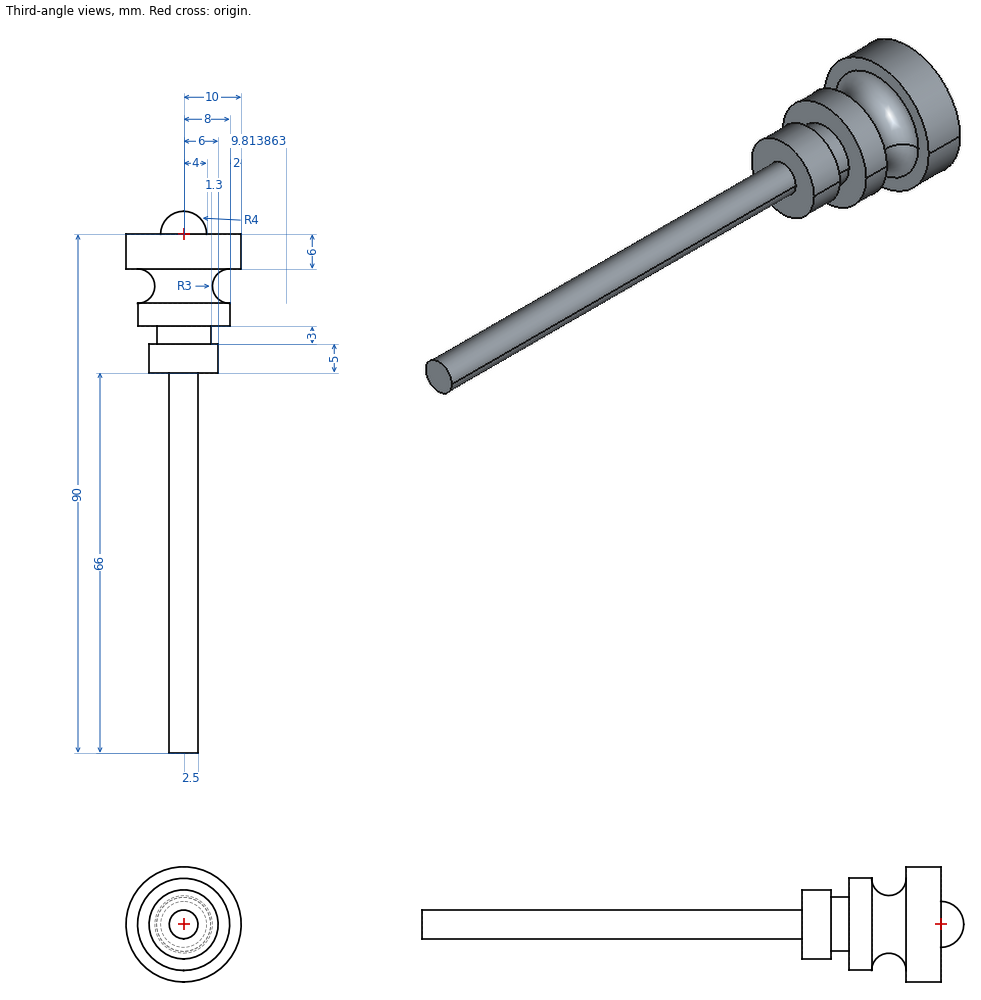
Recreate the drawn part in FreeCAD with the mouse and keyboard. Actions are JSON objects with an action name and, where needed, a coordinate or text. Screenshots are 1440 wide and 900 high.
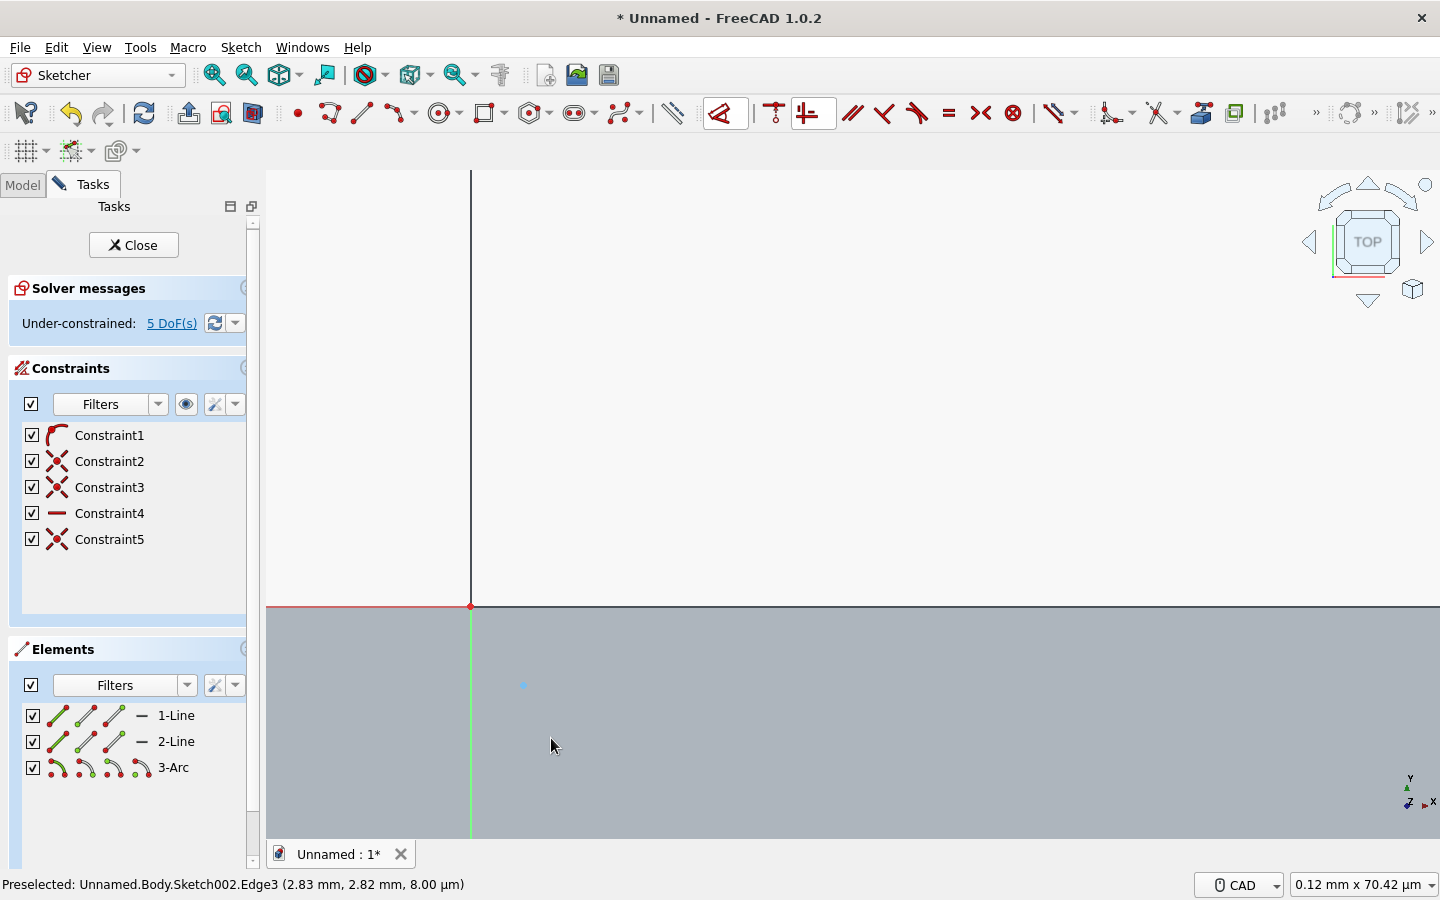
{"action": "left_click_drag", "start_coordinate": [461, 597], "coordinate": [533, 695]}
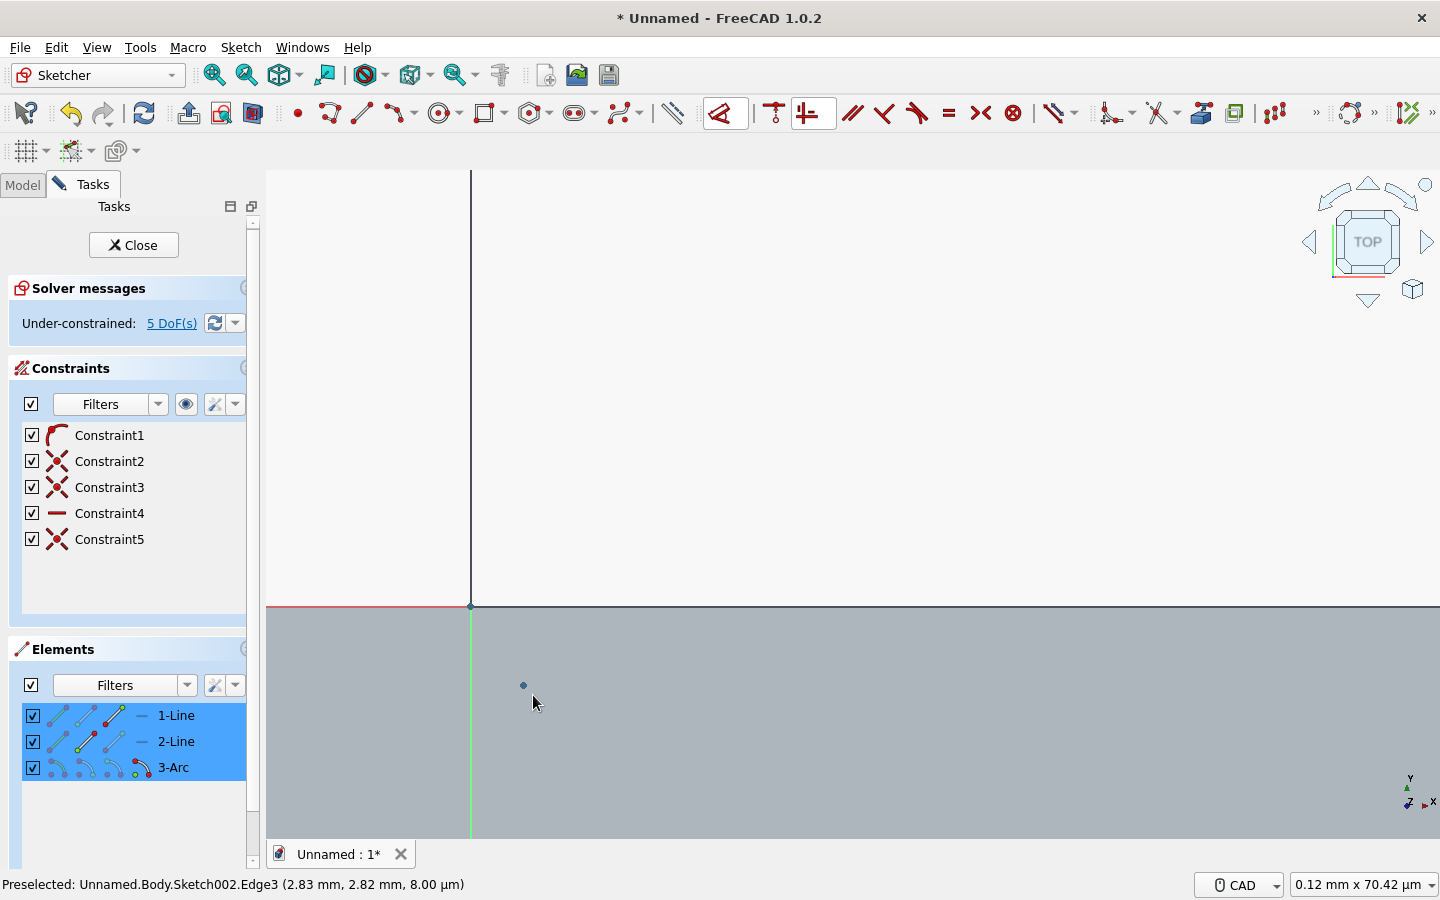
{"action": "key", "text": "c"}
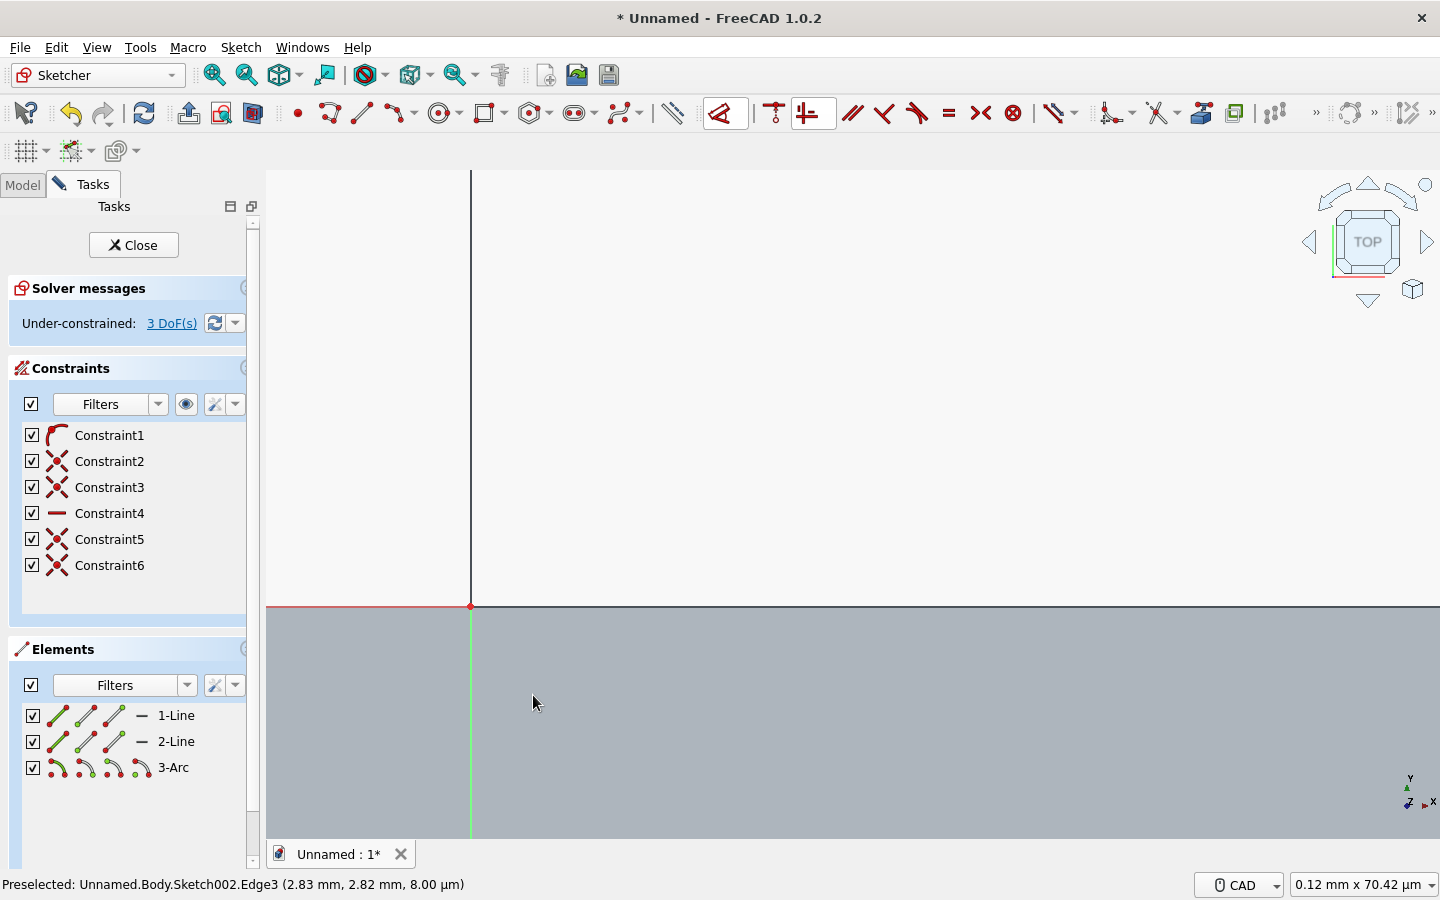
{"action": "scroll", "coordinate": [784, 504], "scroll_direction": "down", "scroll_amount": 15}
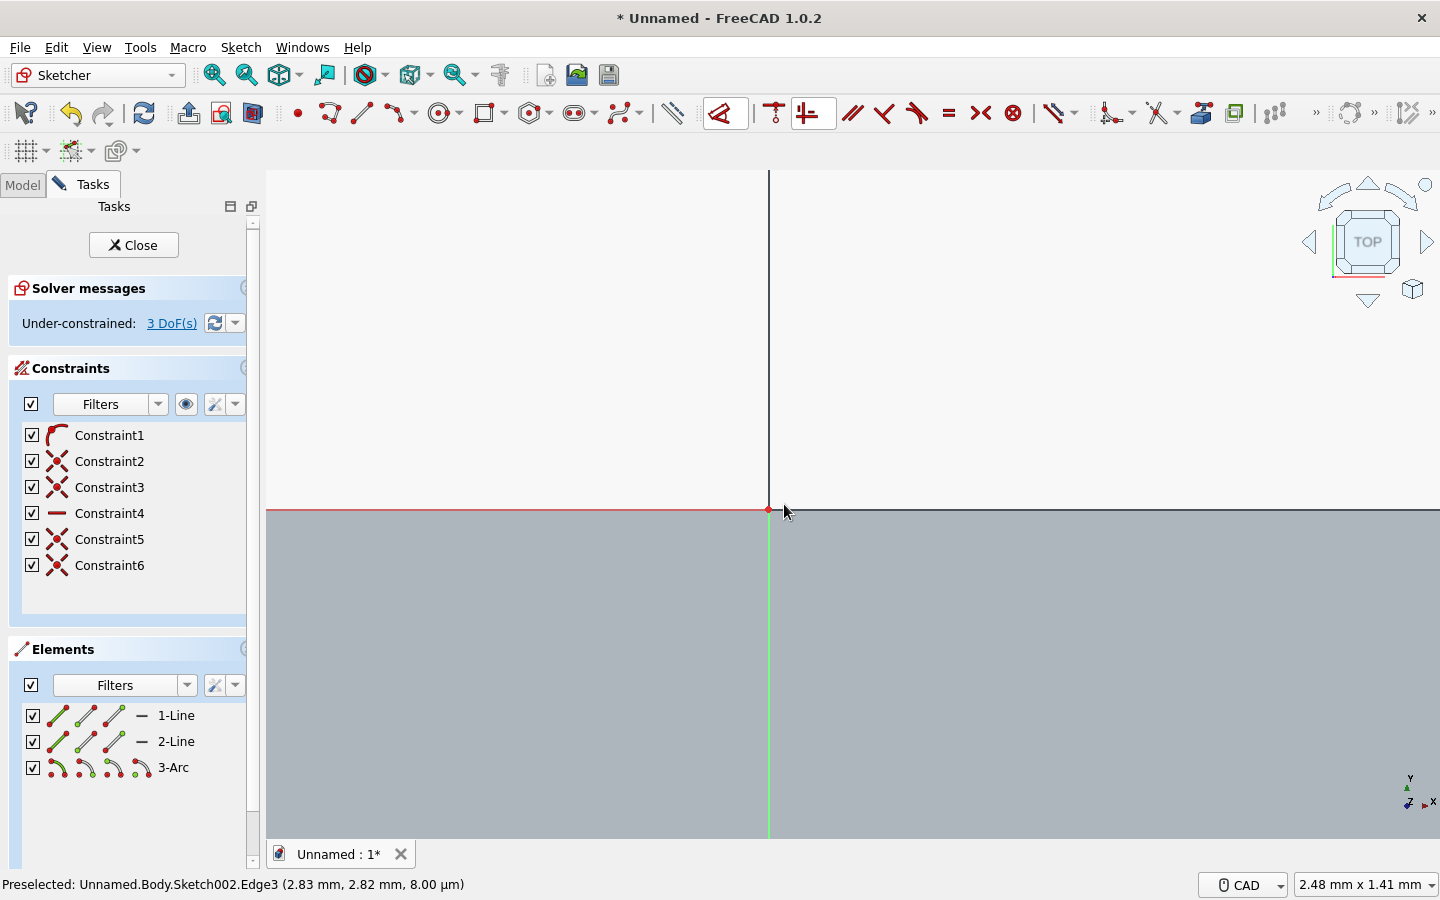
{"action": "scroll", "coordinate": [480, 811], "scroll_direction": "down", "scroll_amount": 7}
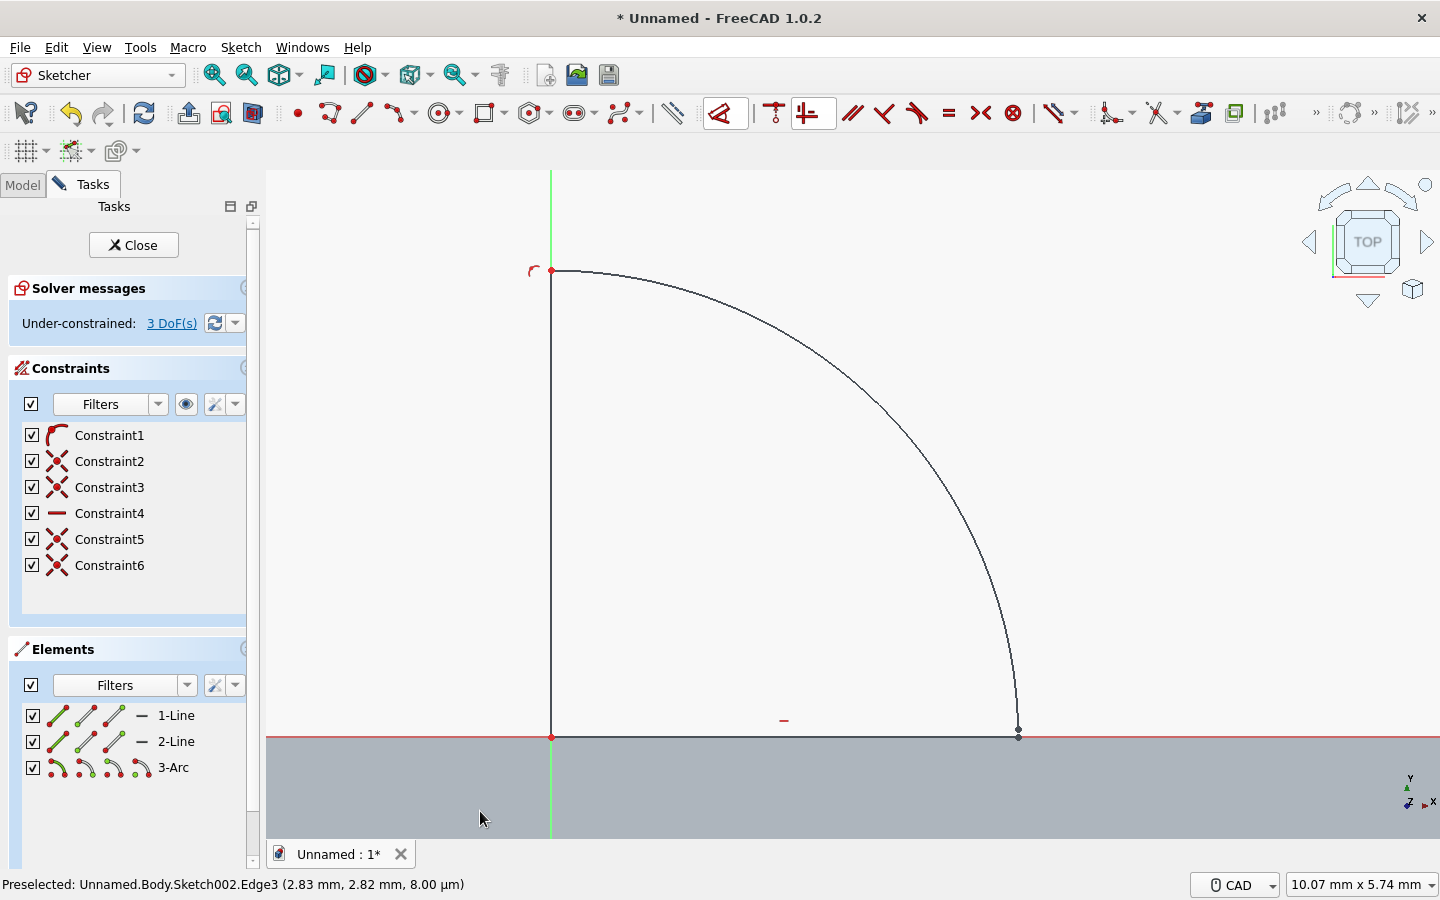
{"action": "left_click", "coordinate": [965, 520]}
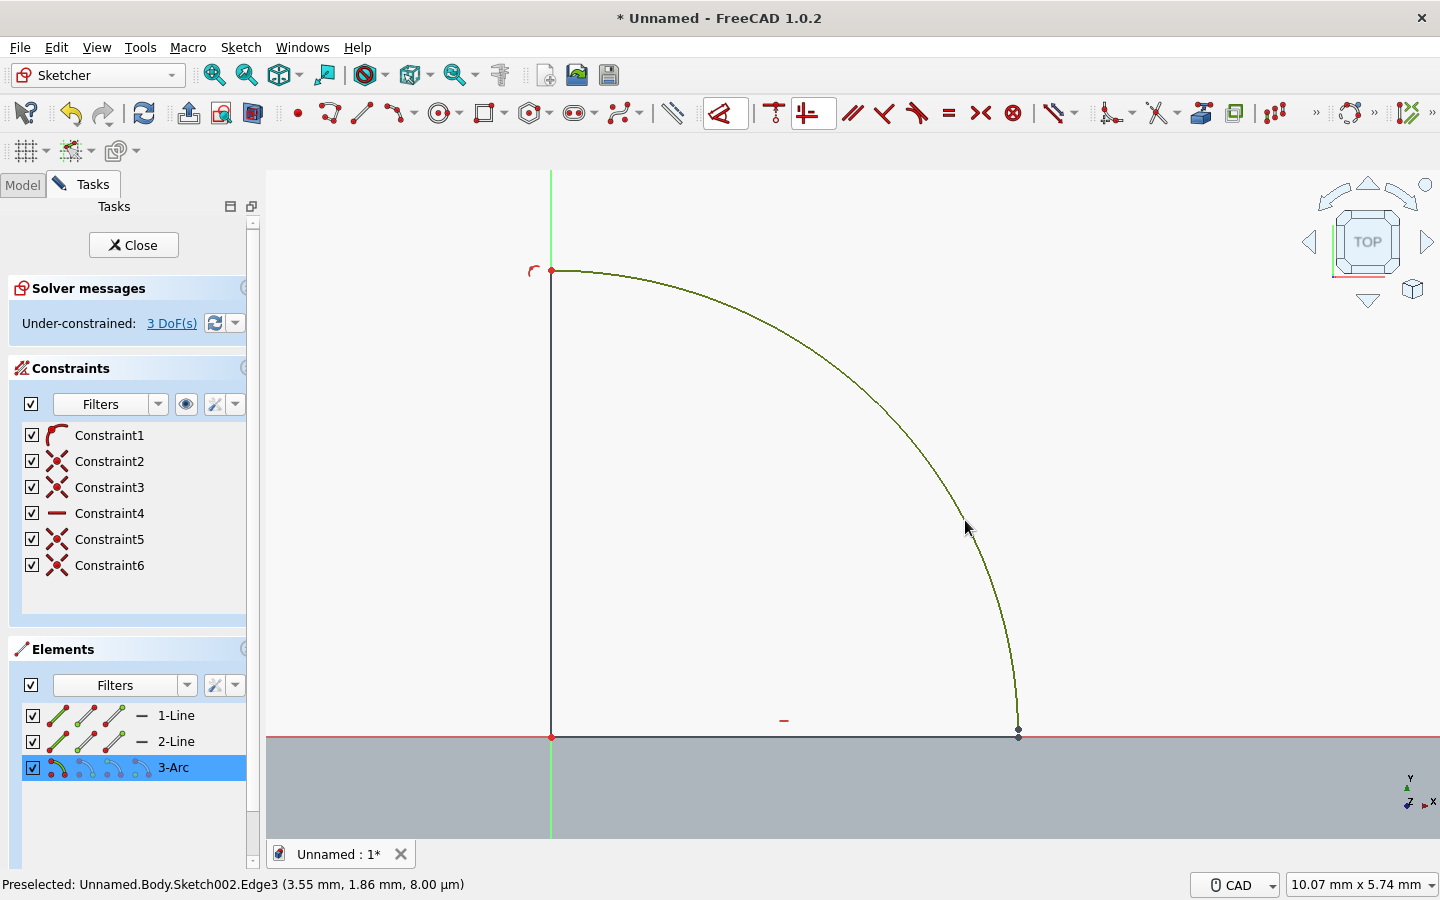
{"action": "left_click", "coordinate": [742, 114]}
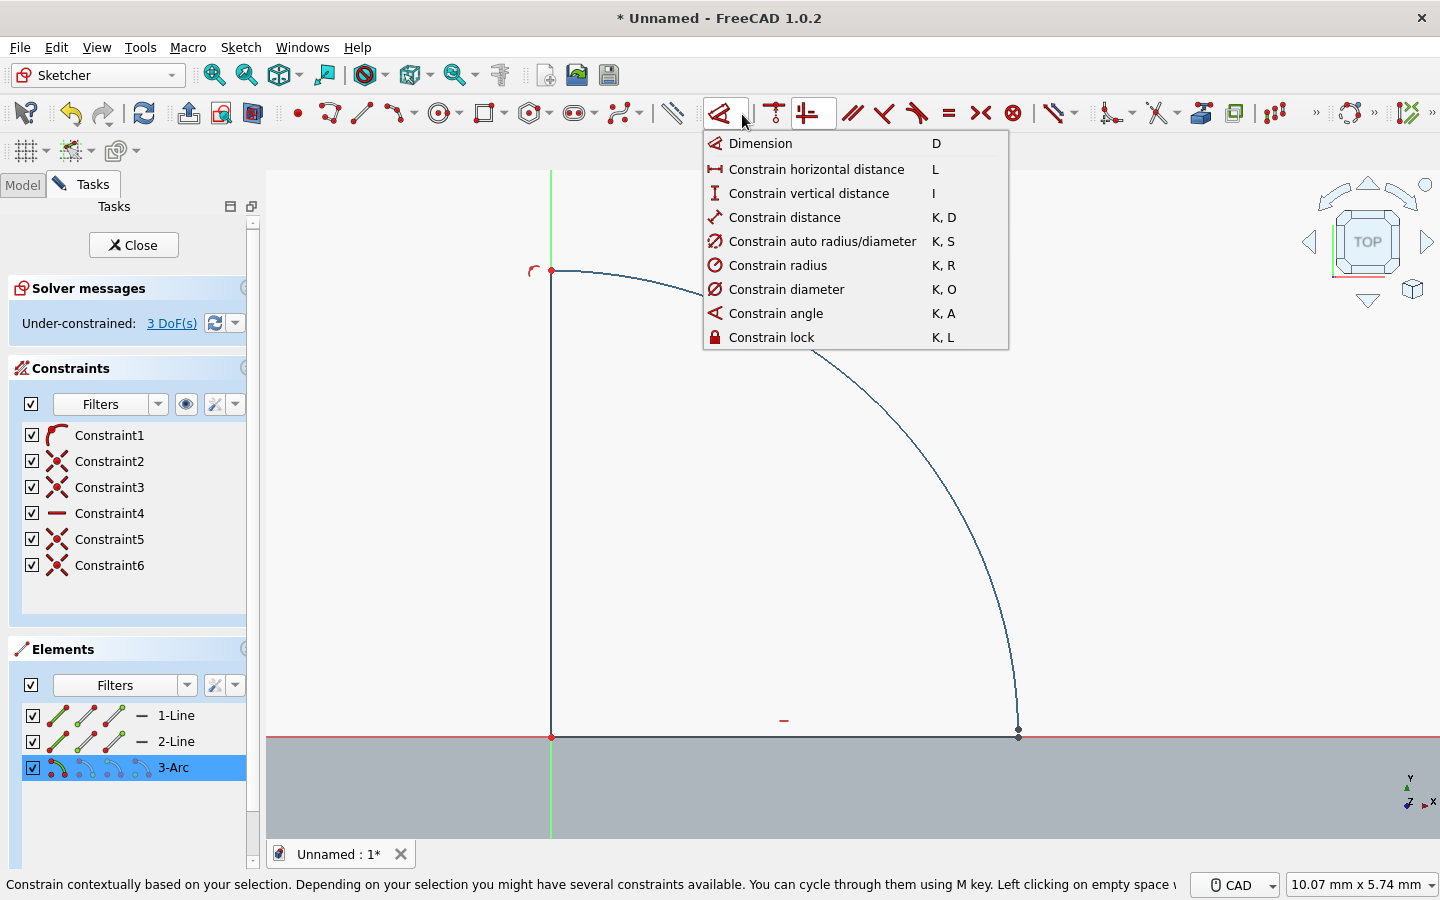
{"action": "left_click", "coordinate": [856, 265]}